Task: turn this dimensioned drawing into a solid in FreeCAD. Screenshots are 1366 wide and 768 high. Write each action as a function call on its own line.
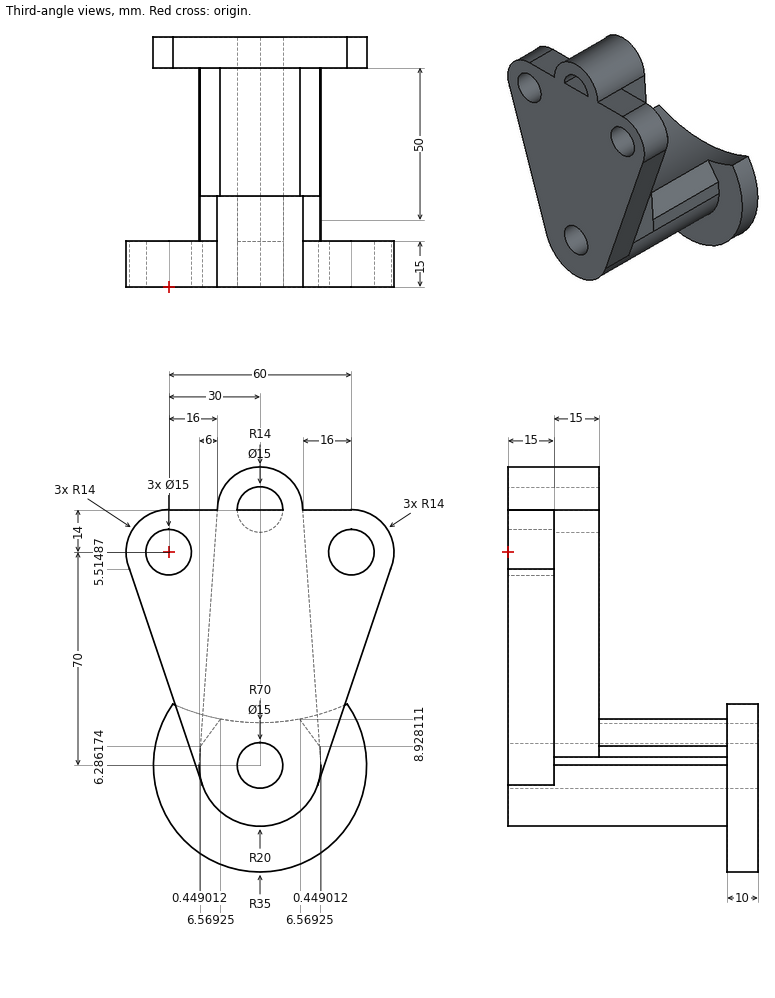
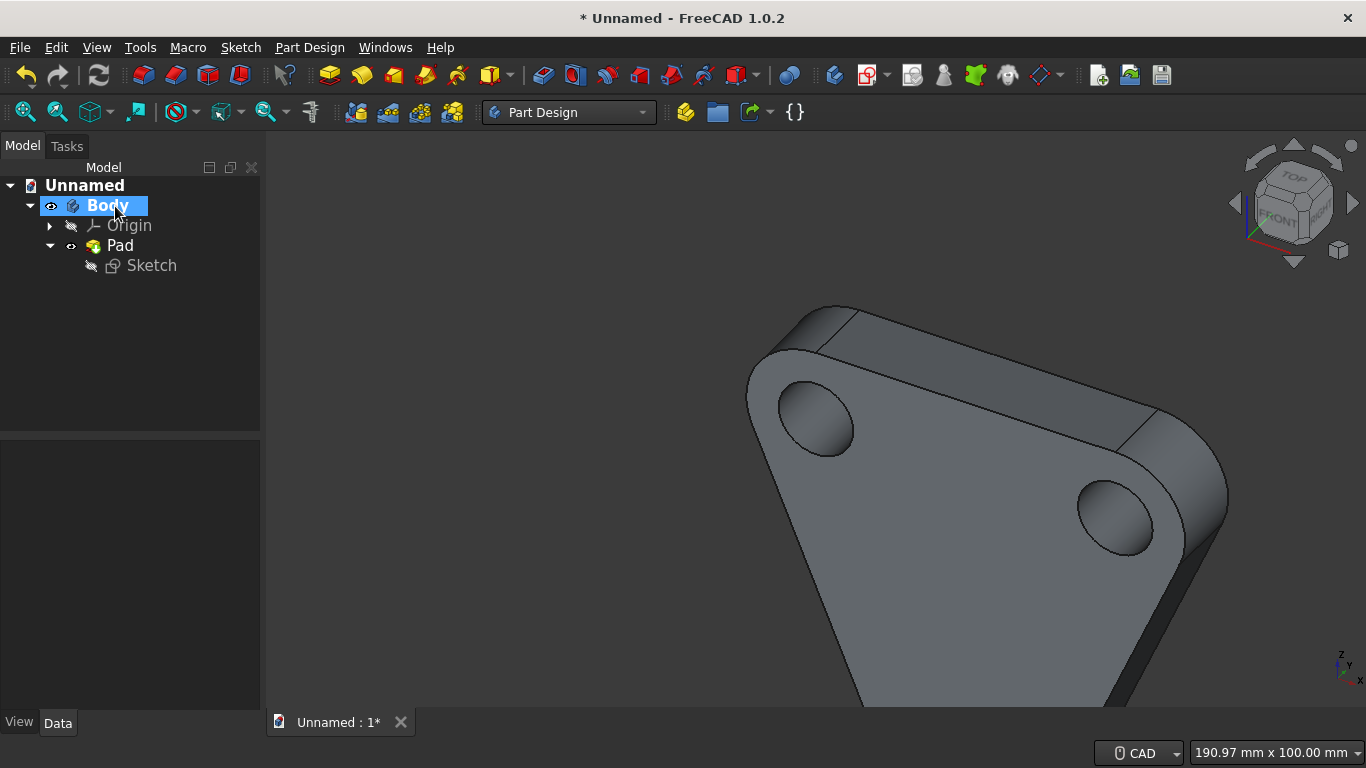
click(26, 112)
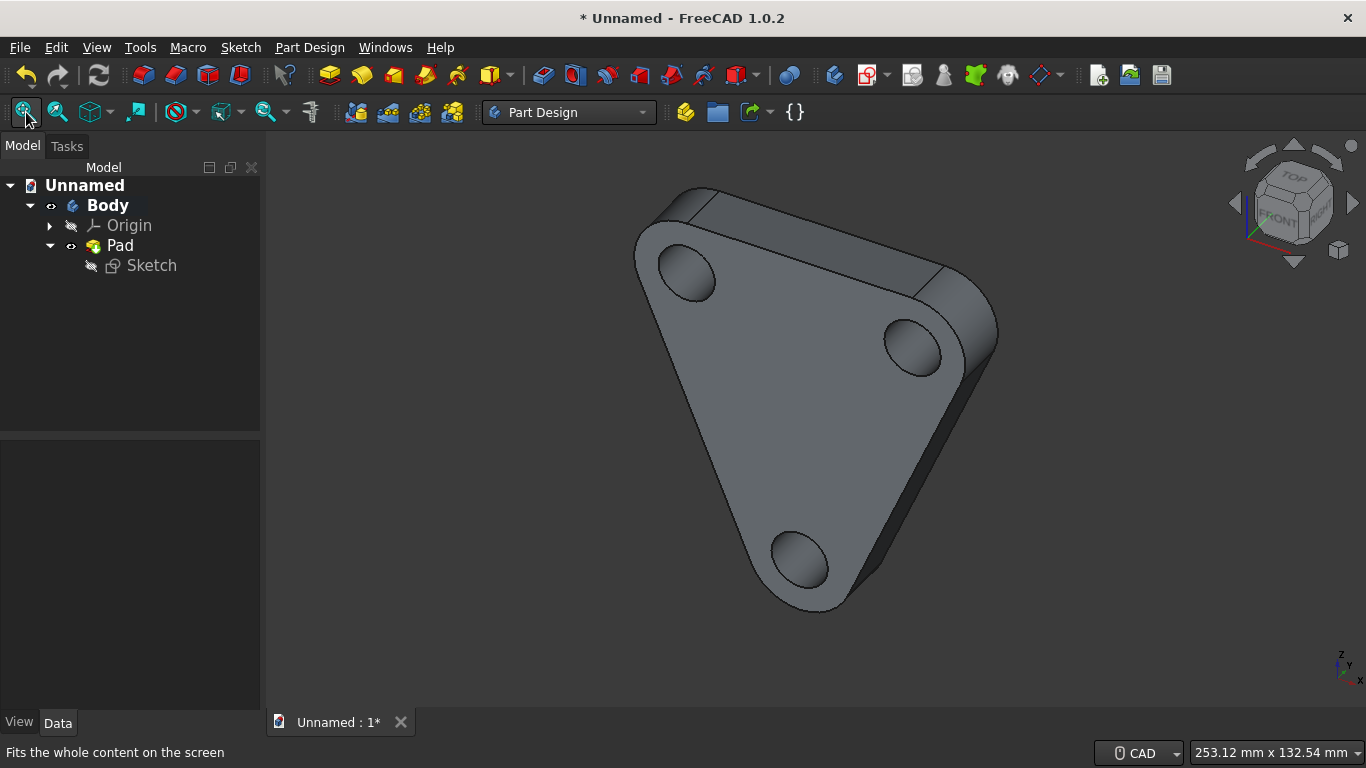
click(800, 384)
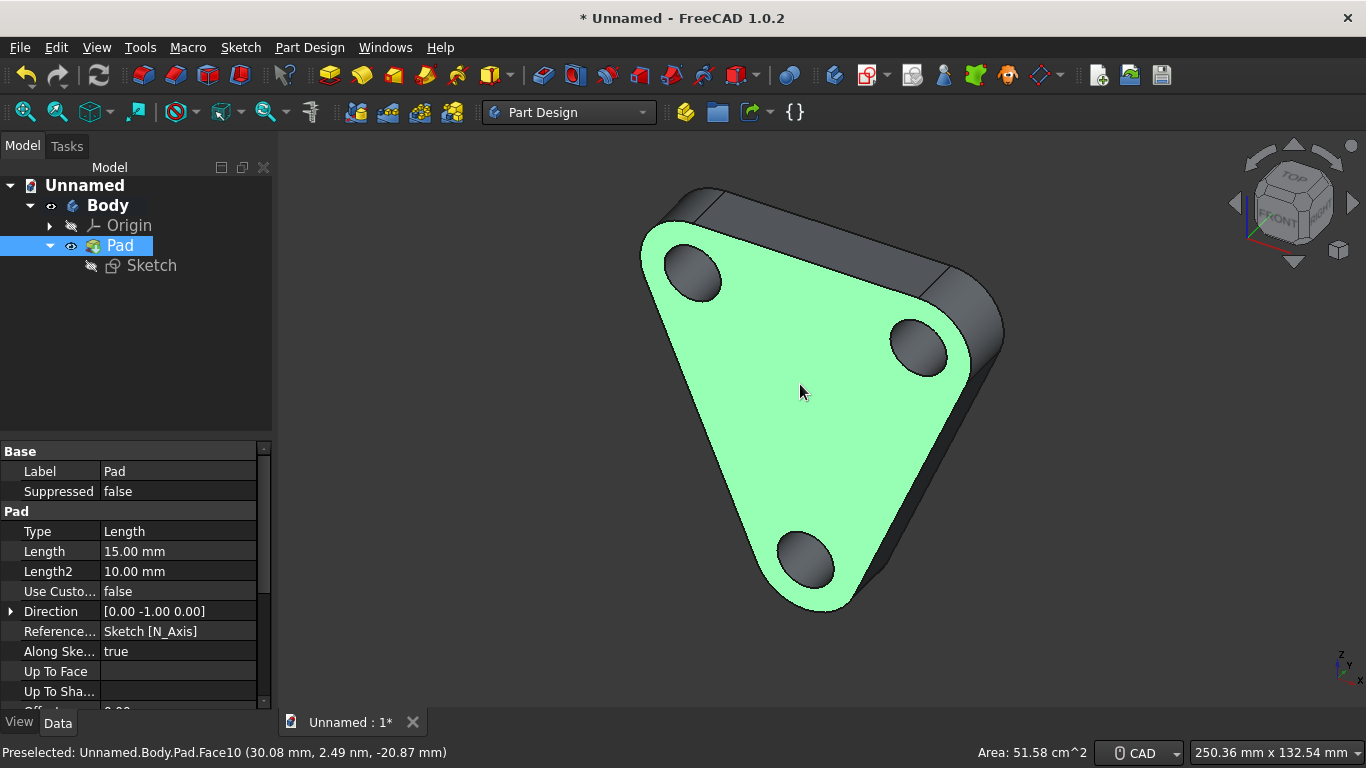
click(868, 76)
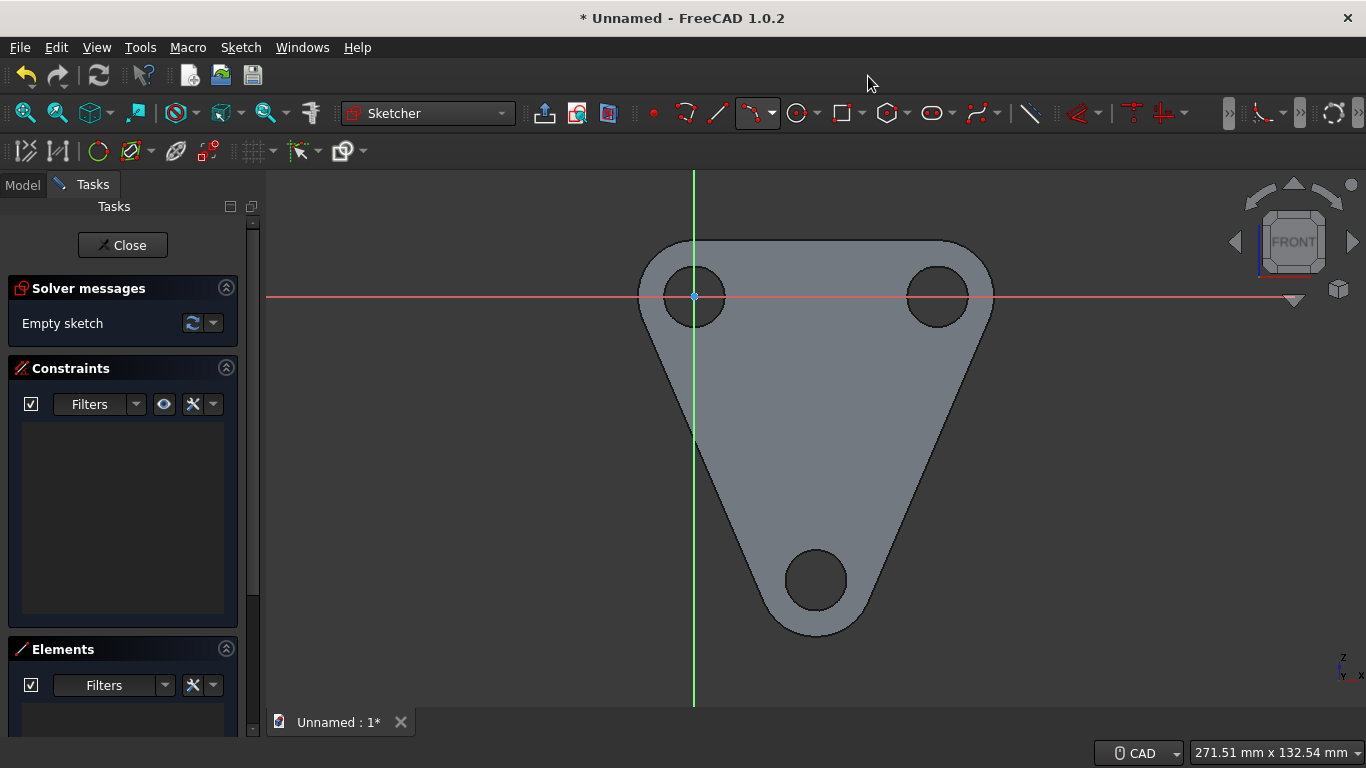
scroll(608, 471, down, 2)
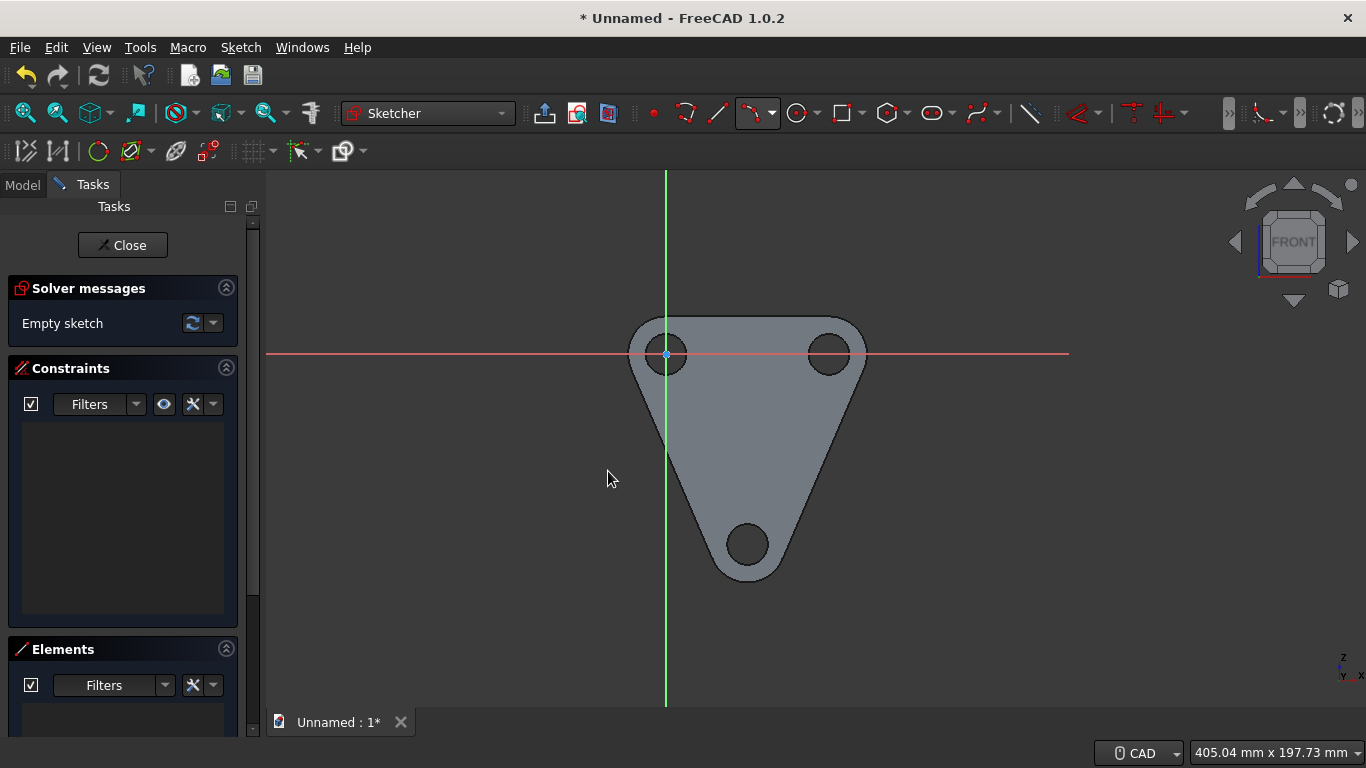
click(718, 114)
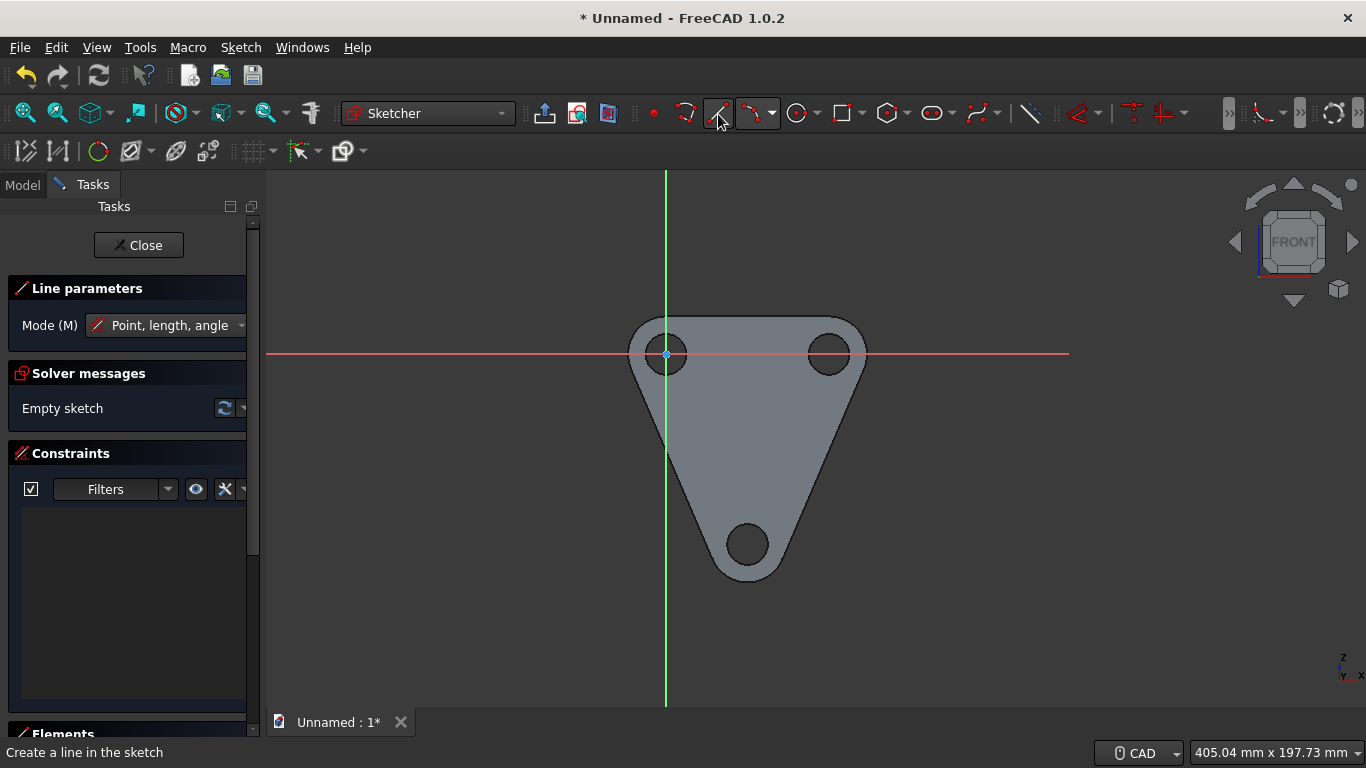
click(631, 369)
click(696, 562)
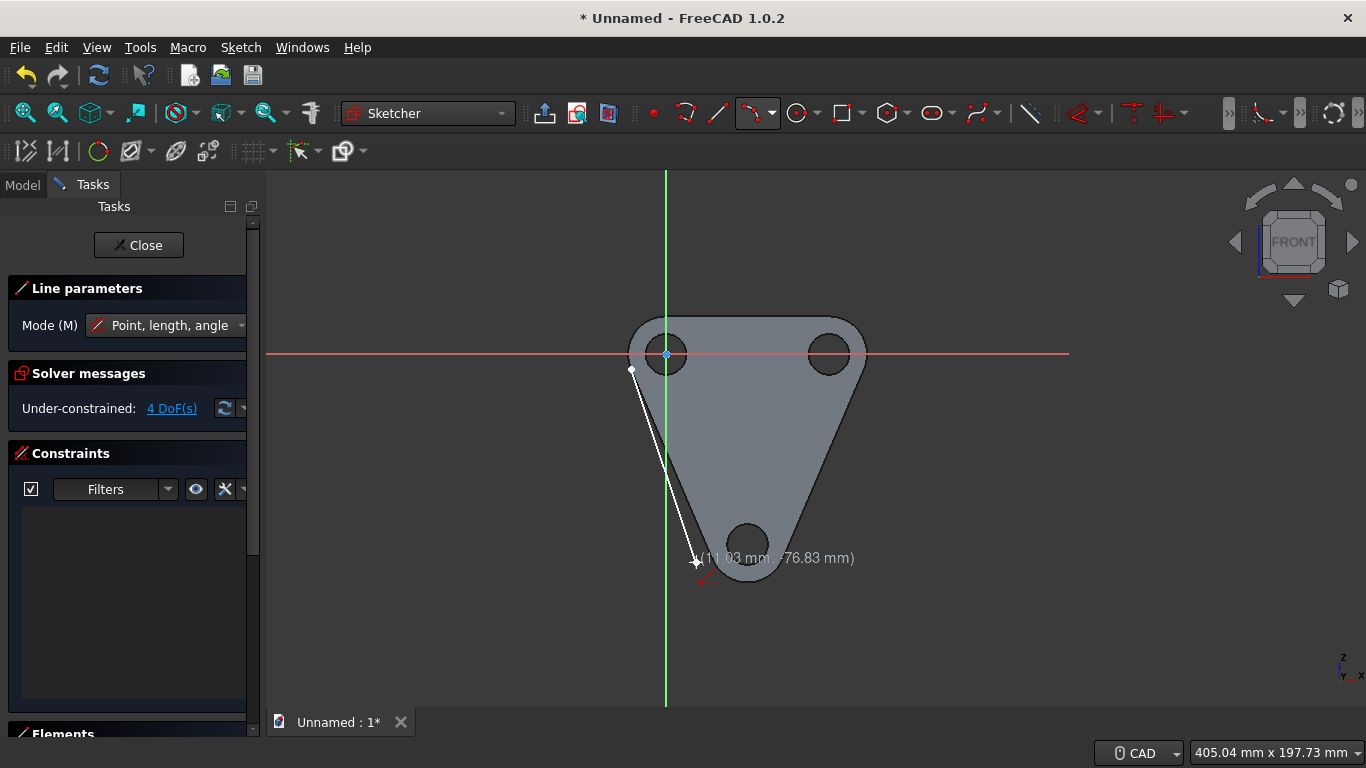
click(799, 562)
click(864, 369)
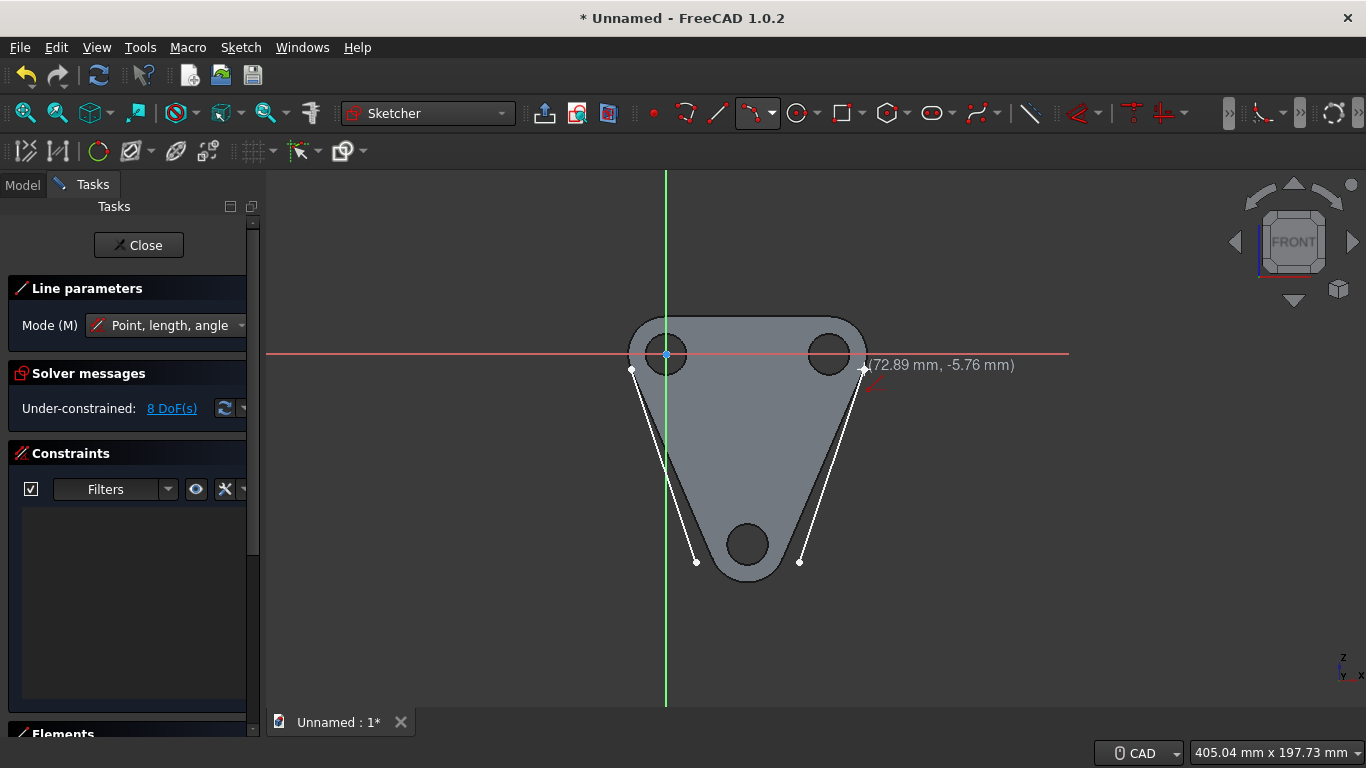
click(829, 316)
click(786, 316)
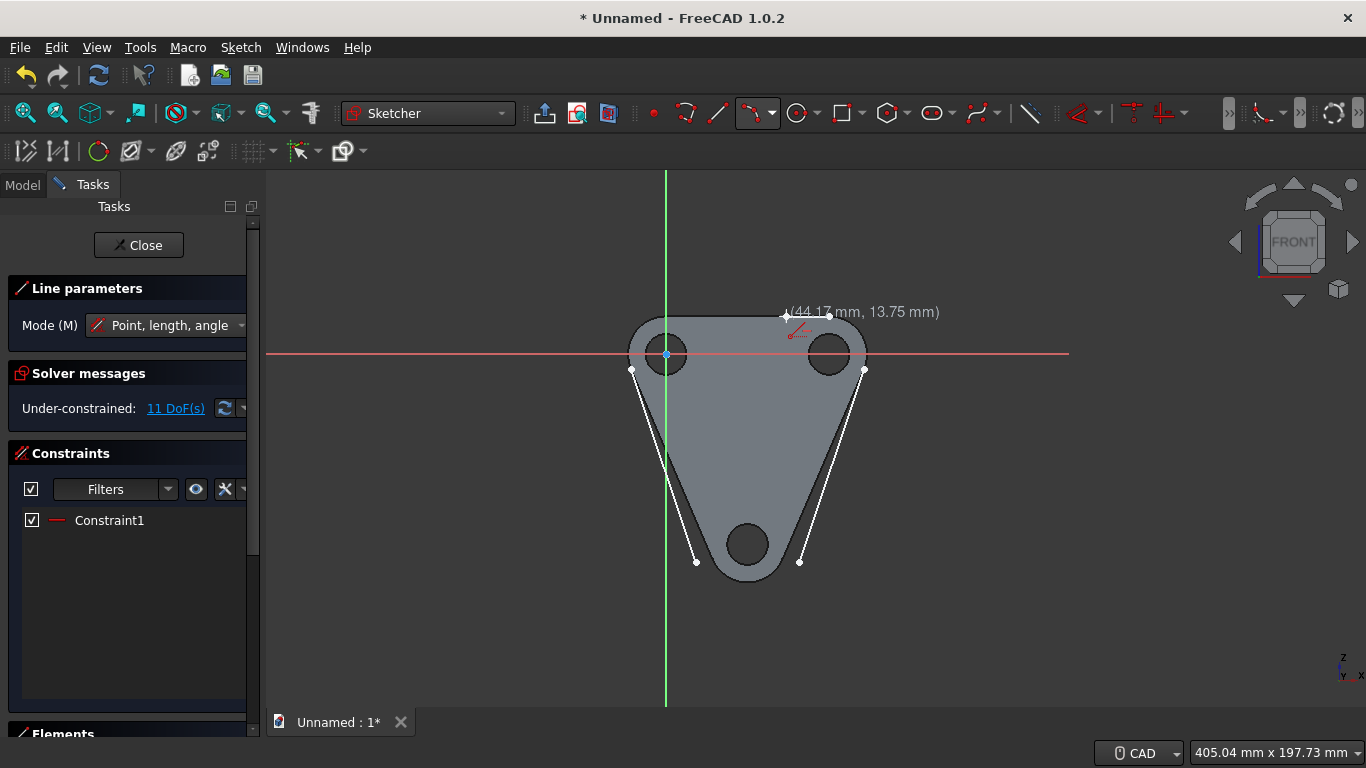
click(710, 316)
click(666, 316)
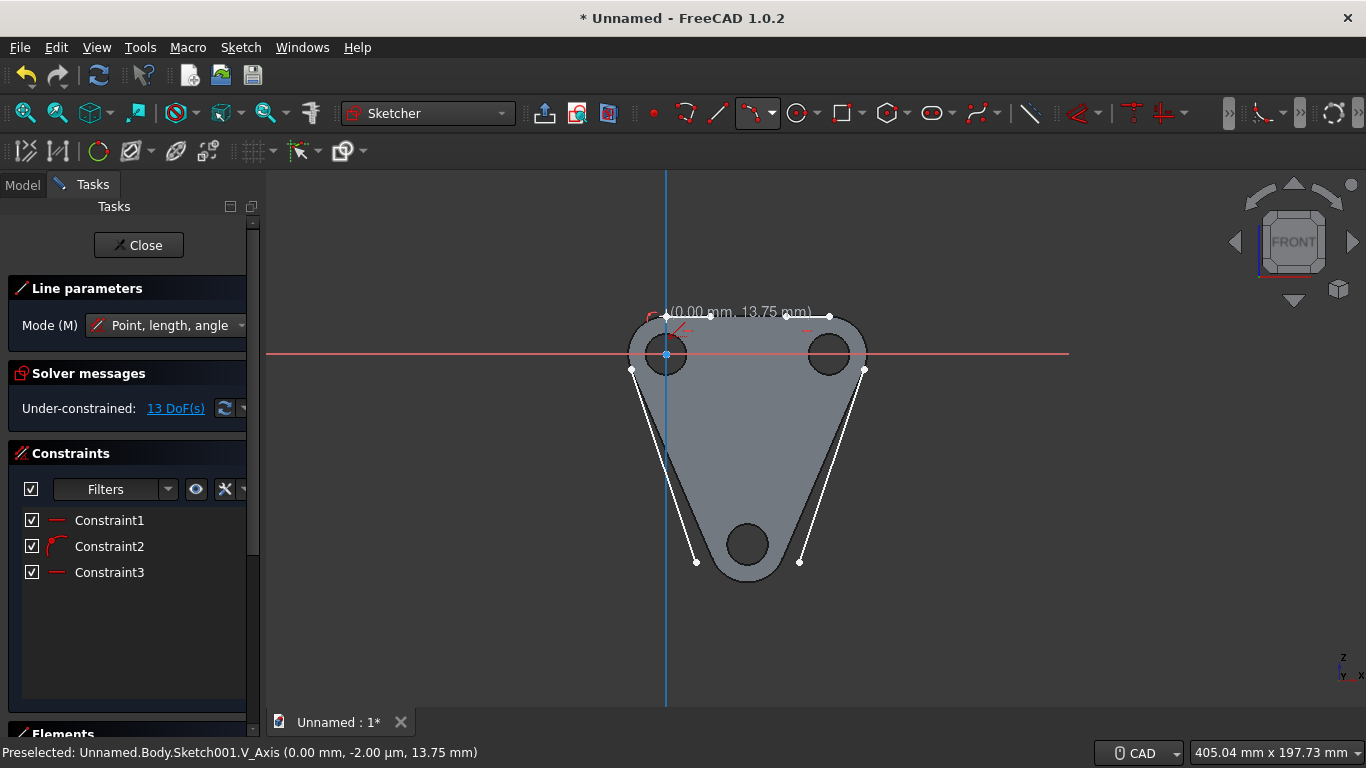
click(752, 114)